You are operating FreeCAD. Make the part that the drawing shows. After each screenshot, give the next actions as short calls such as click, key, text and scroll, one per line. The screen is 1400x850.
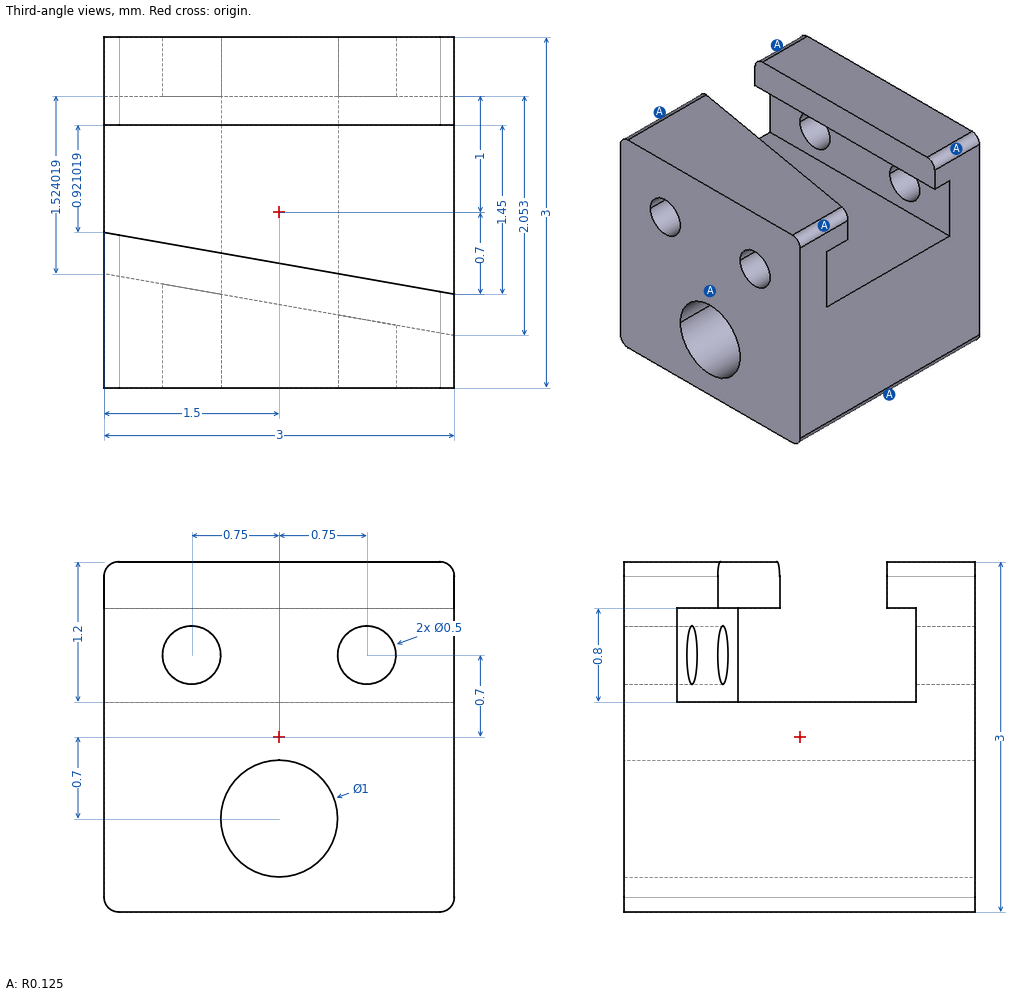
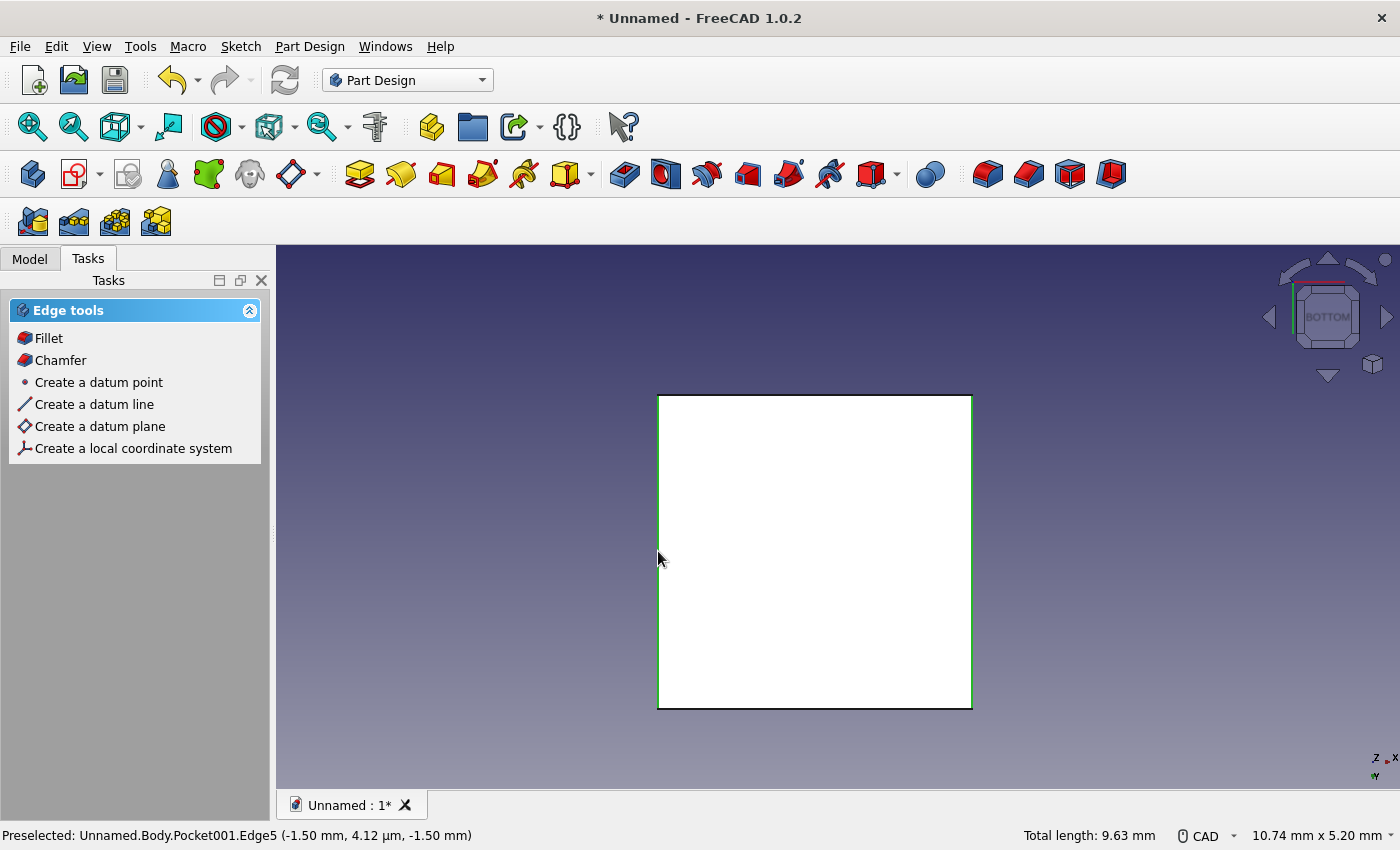
click(988, 174)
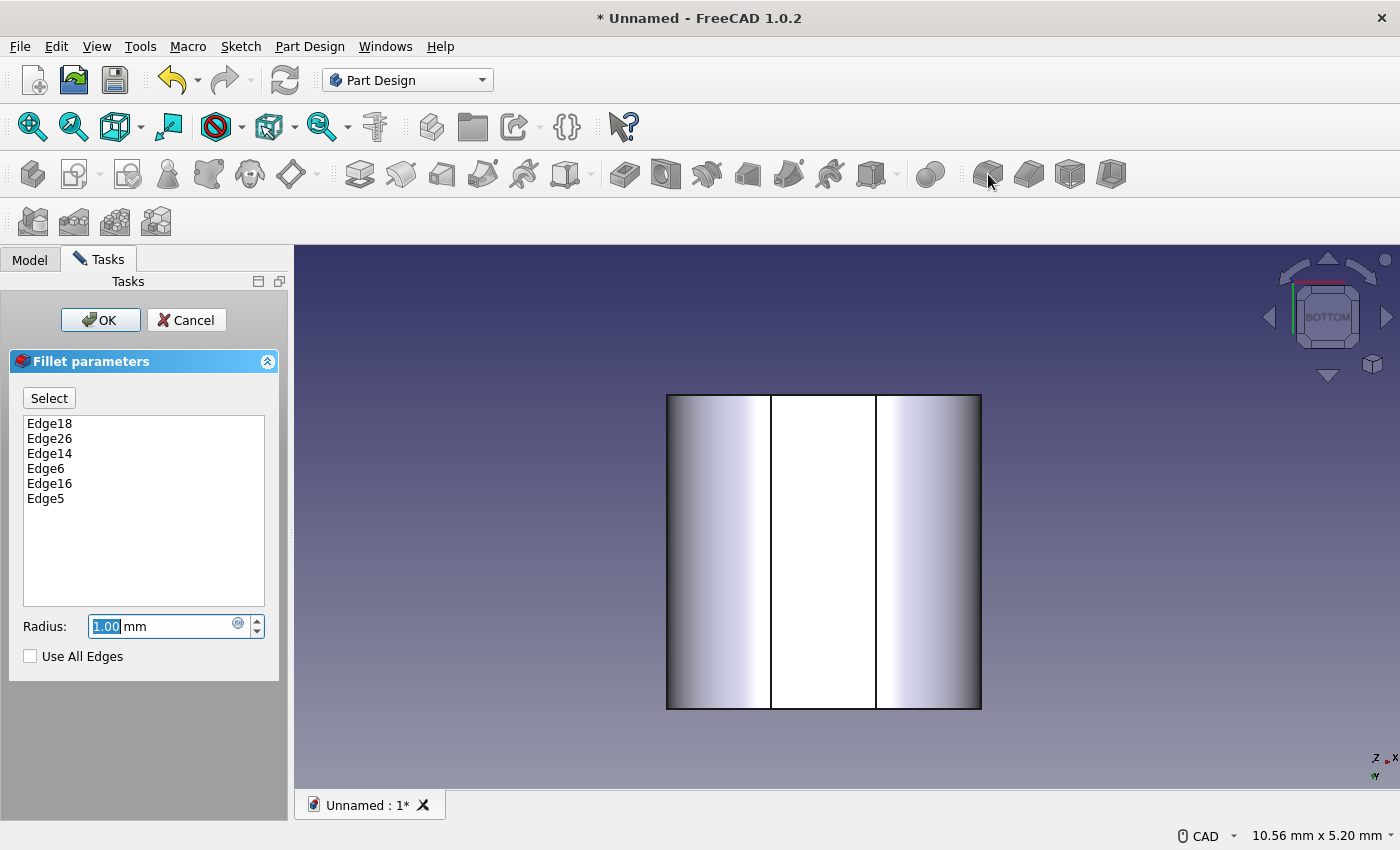
text(0.125)
key(Tab)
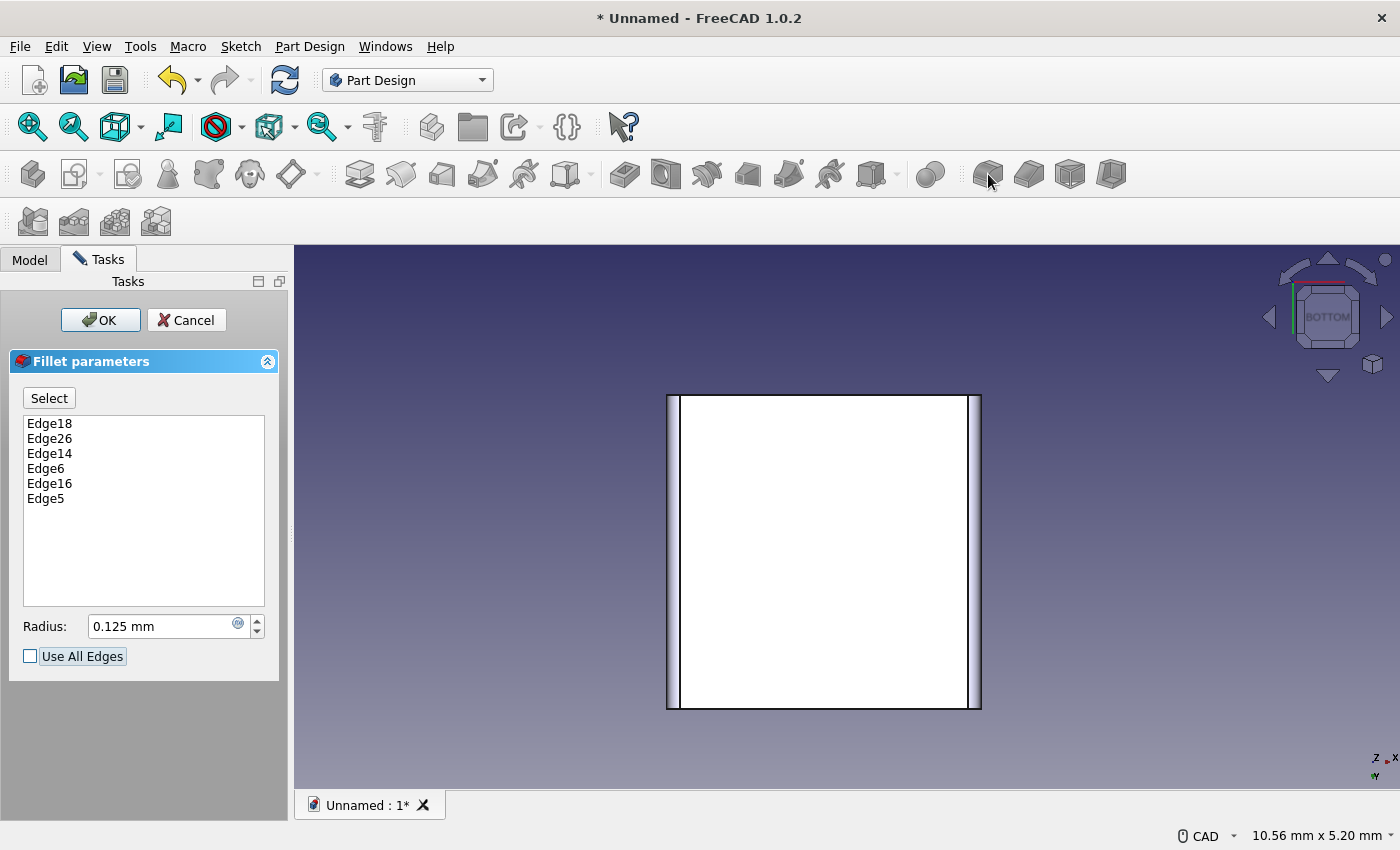
click(101, 320)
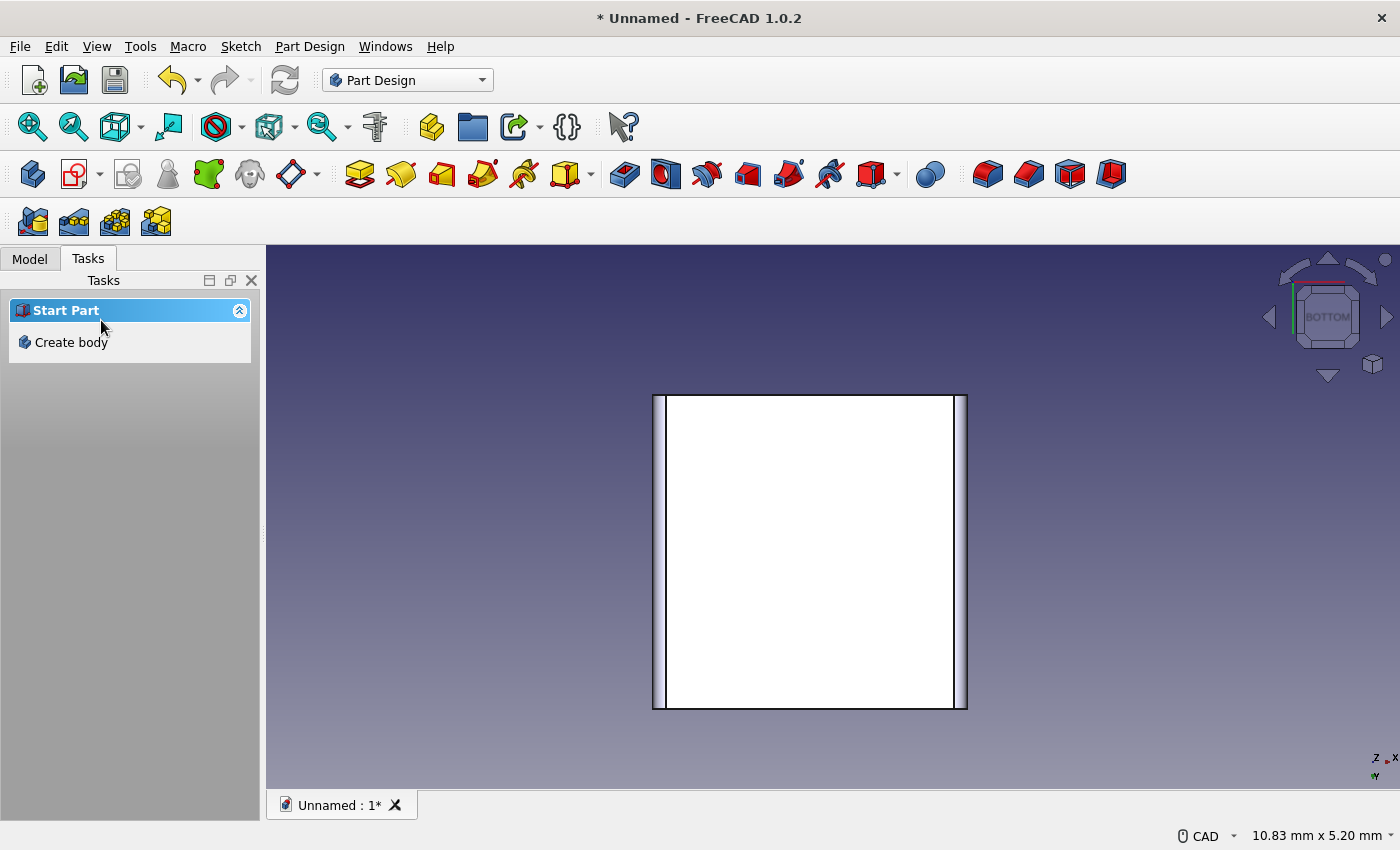
key(4)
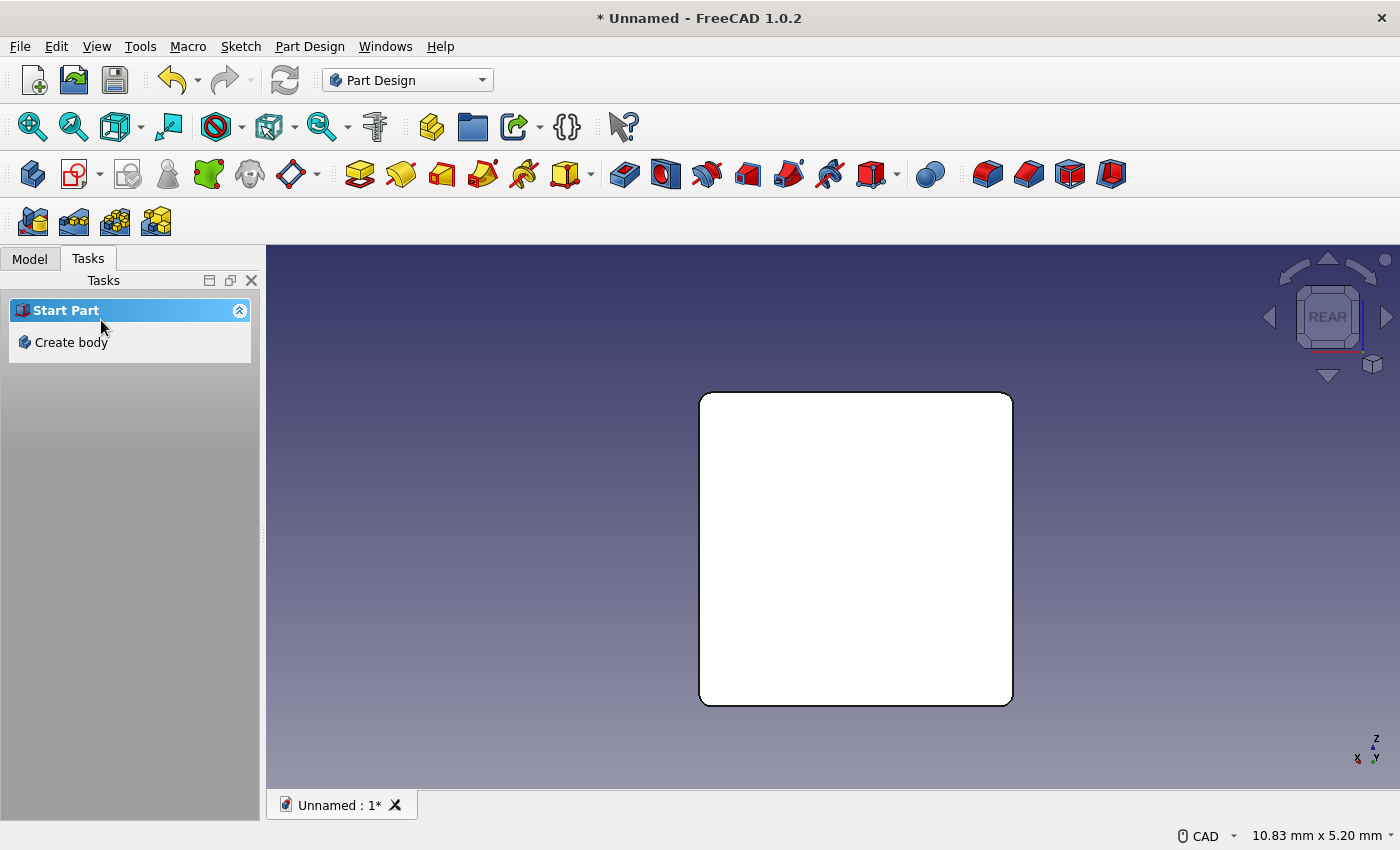
click(856, 548)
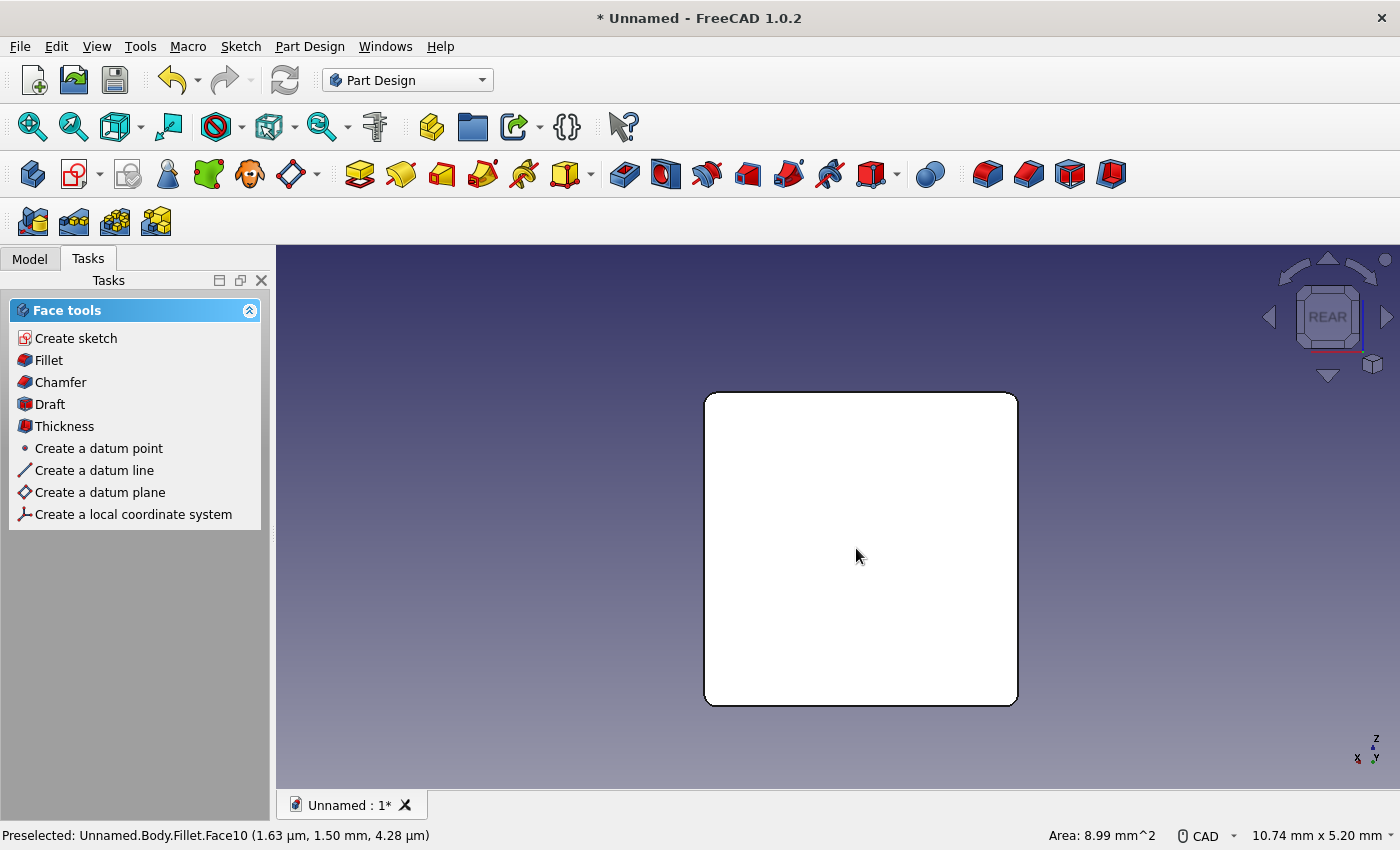
click(74, 174)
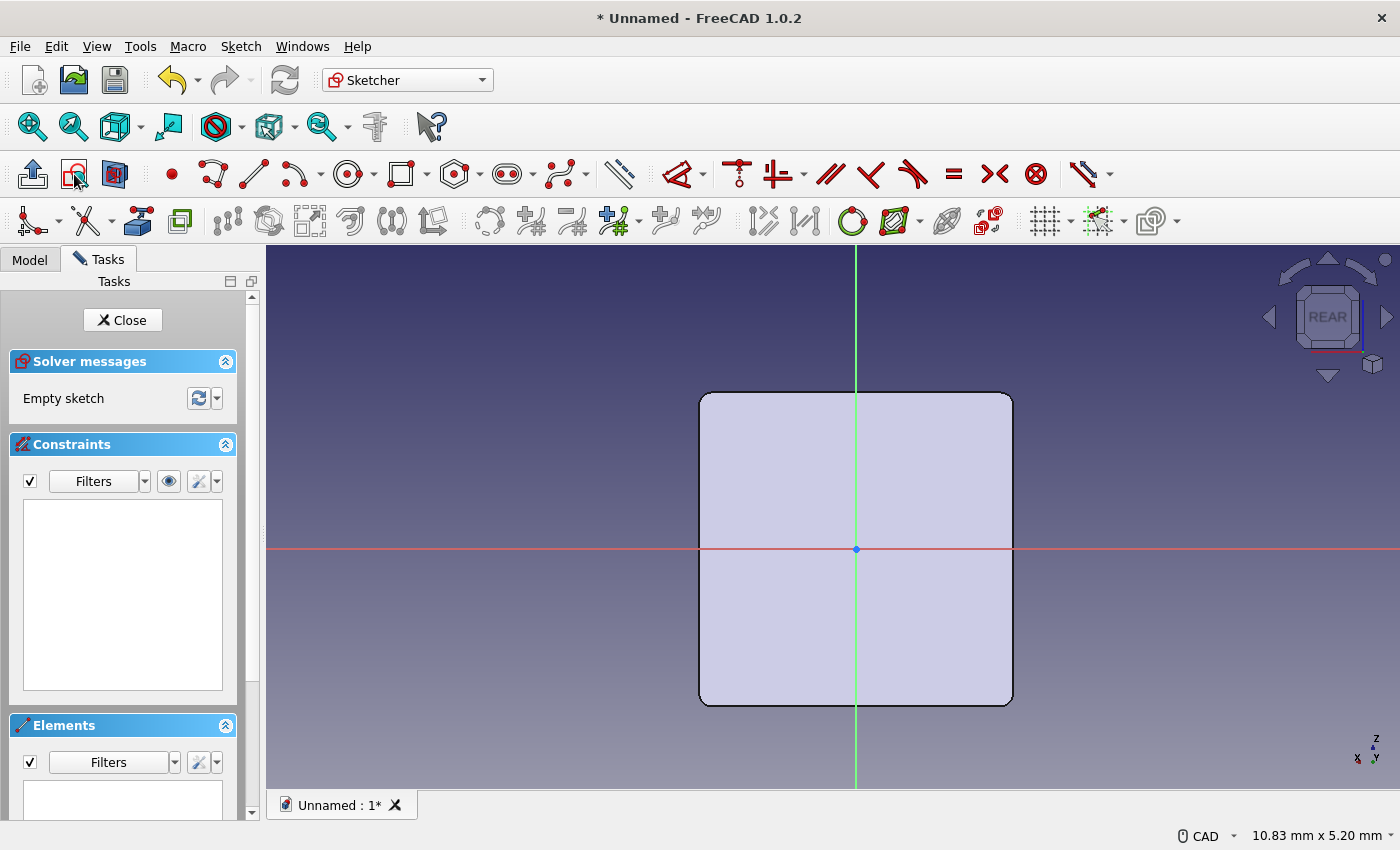
scroll(1043, 655, up, 2)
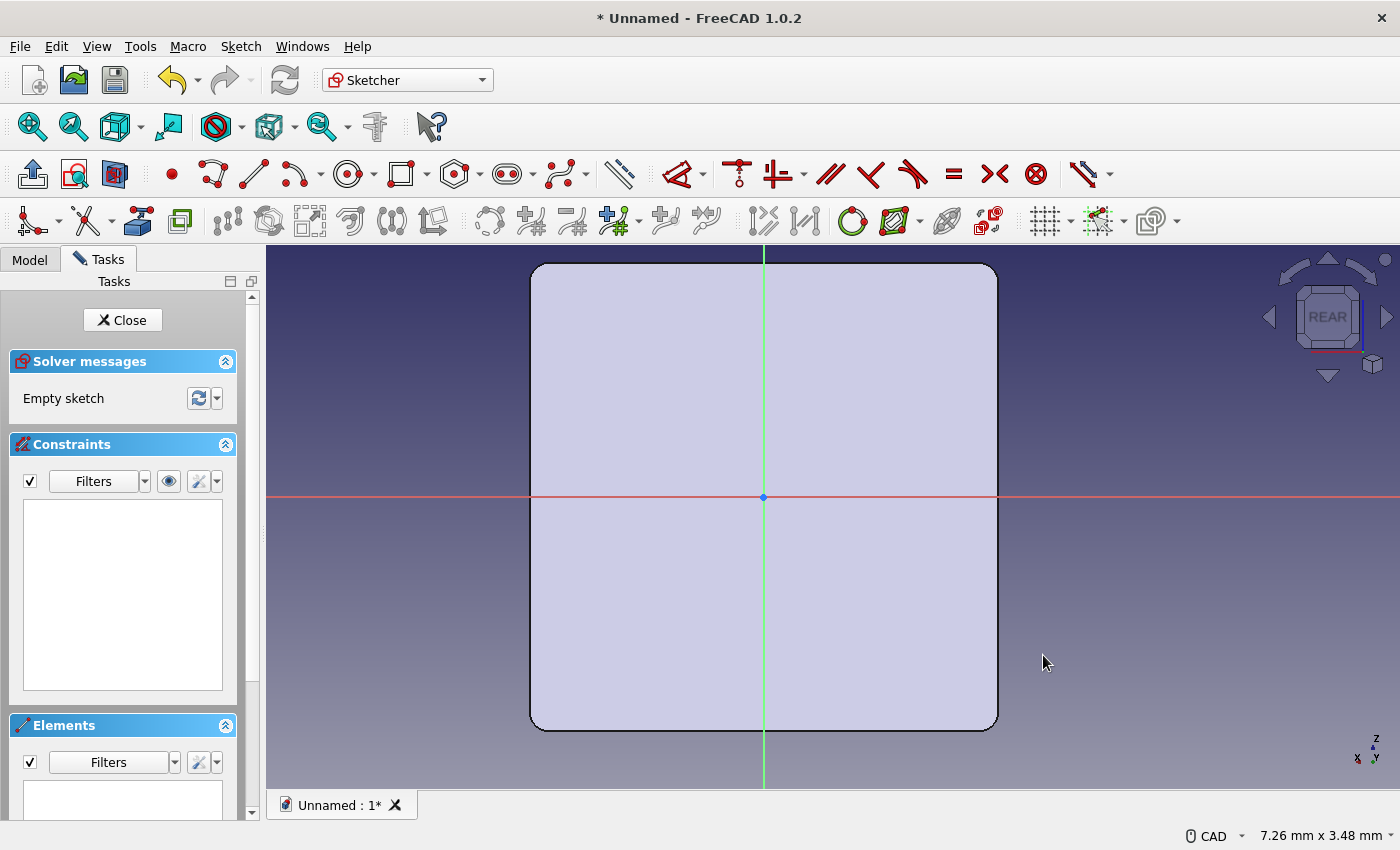
key(g)
key(c)